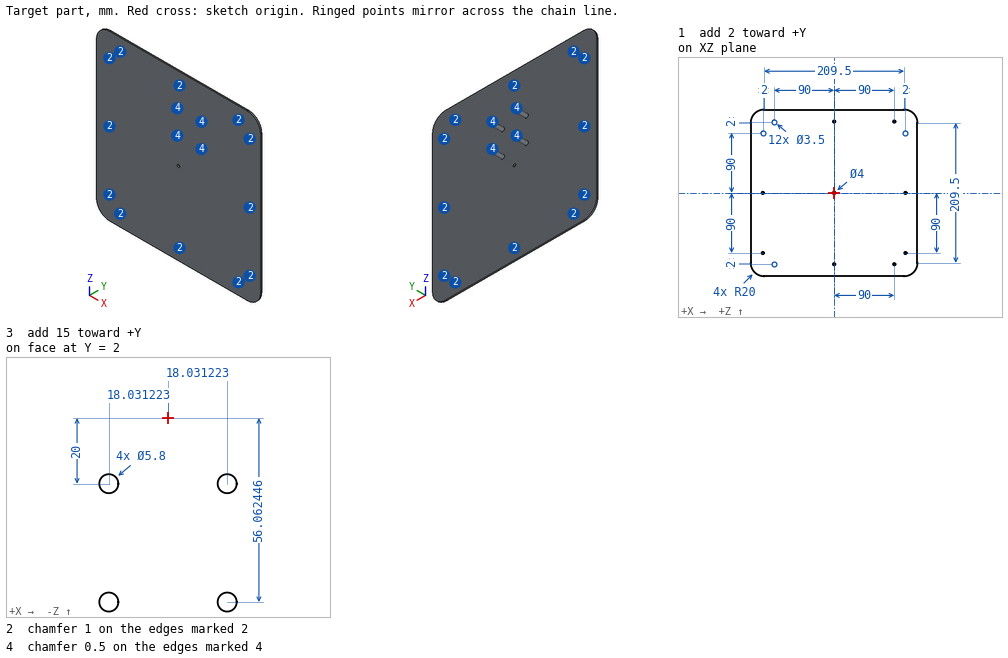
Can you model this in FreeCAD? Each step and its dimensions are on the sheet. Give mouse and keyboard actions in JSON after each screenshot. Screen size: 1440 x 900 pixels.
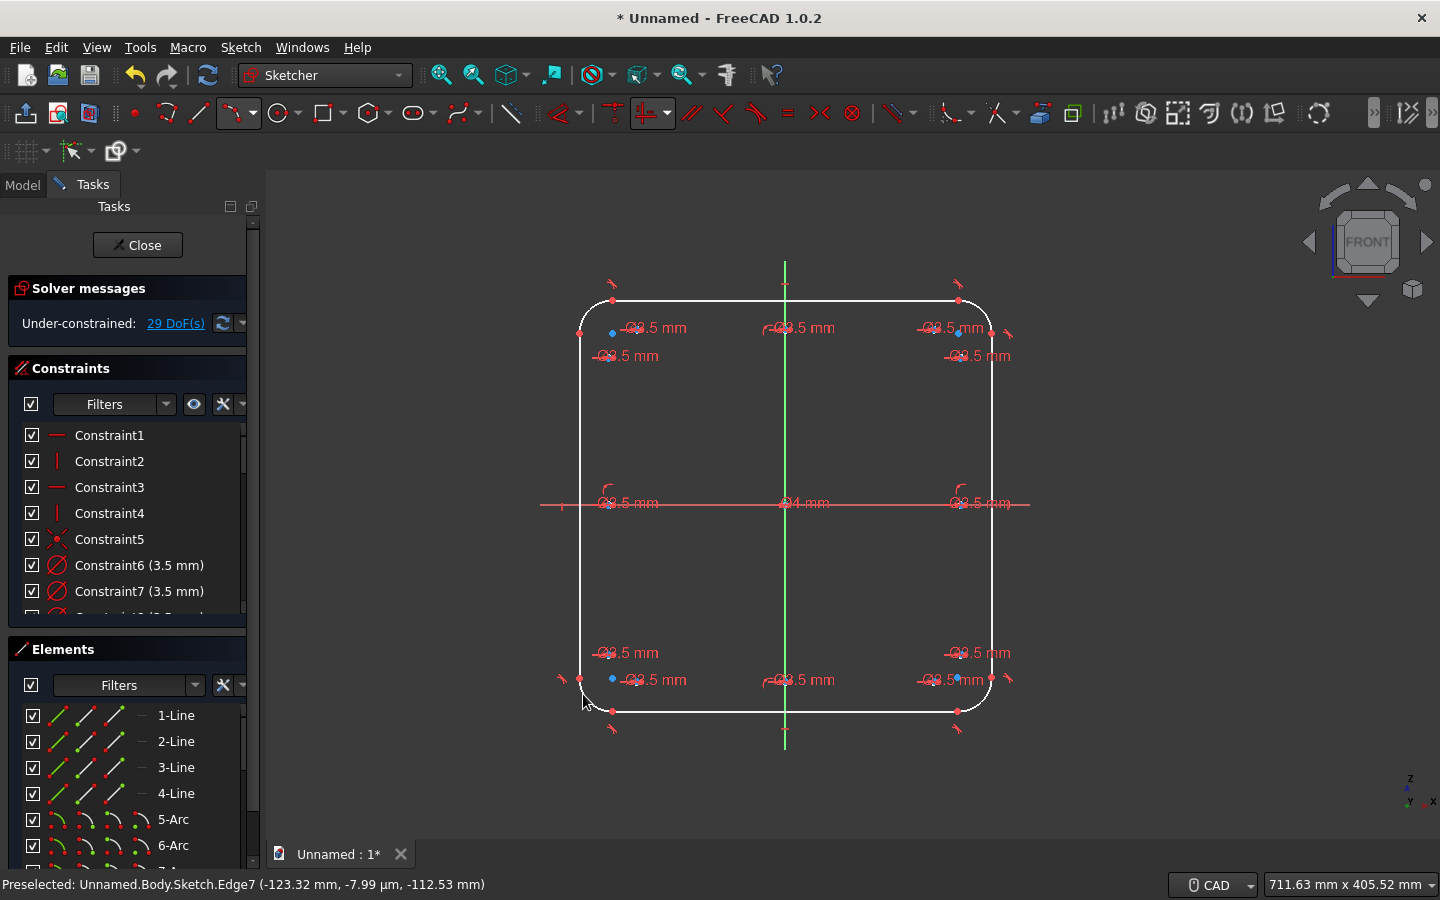
{"action": "left_click", "coordinate": [580, 575]}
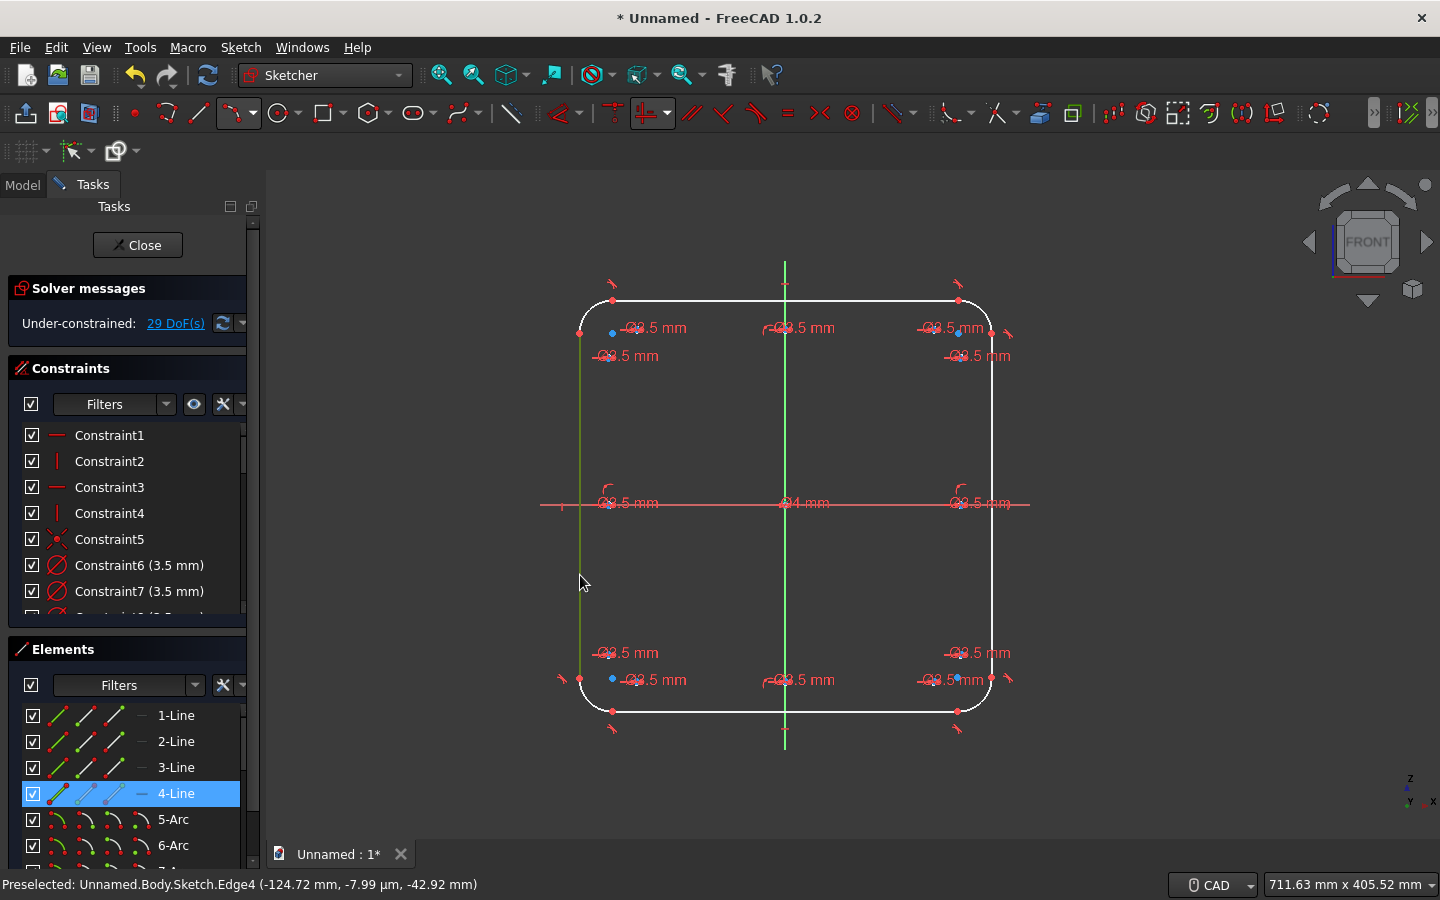
{"action": "left_click", "coordinate": [598, 304]}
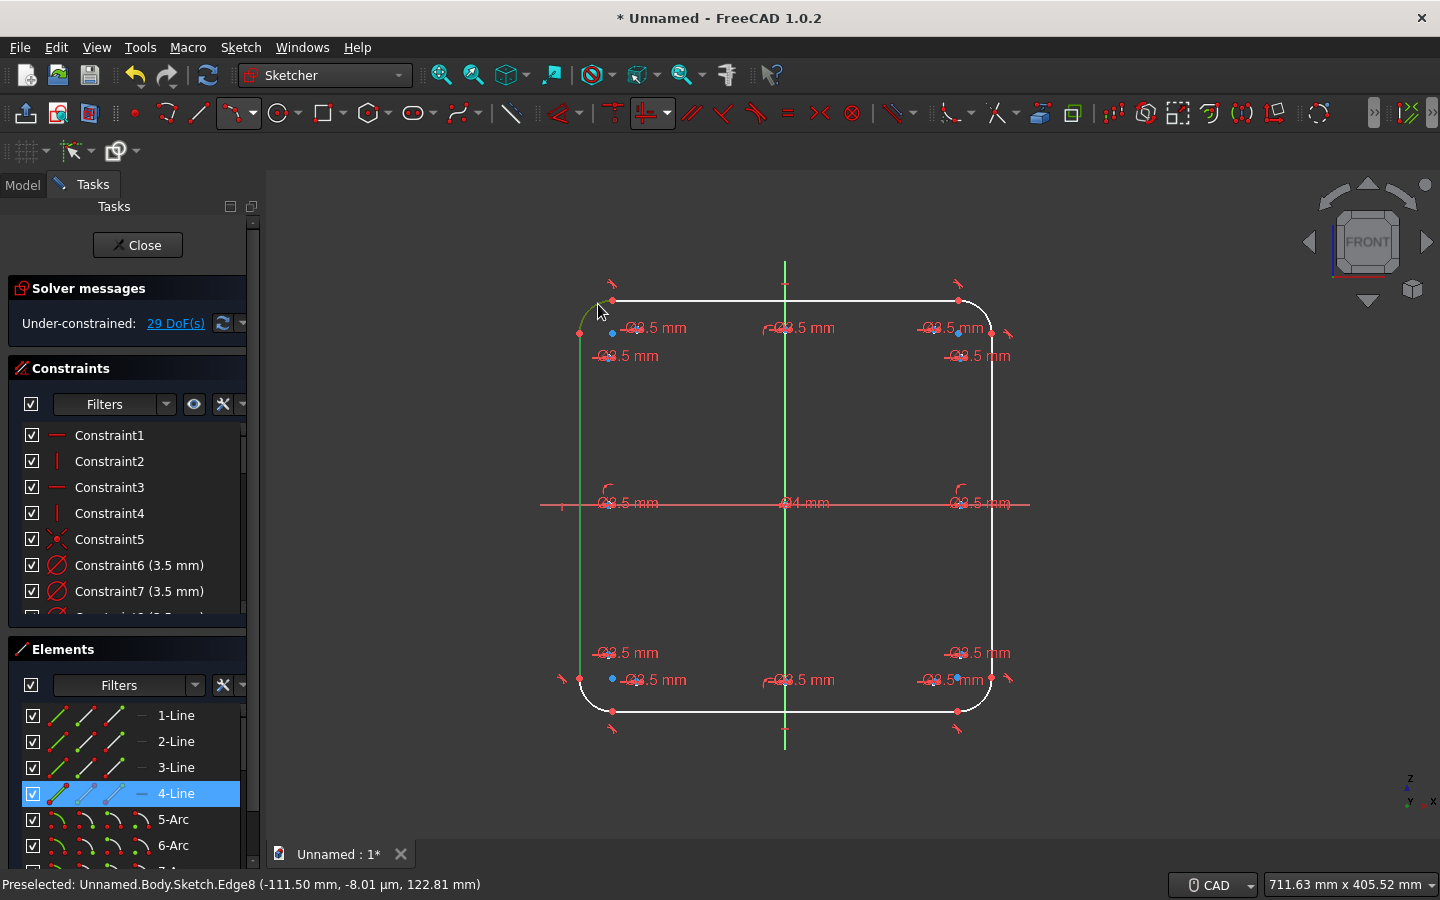
{"action": "left_click", "coordinate": [756, 114]}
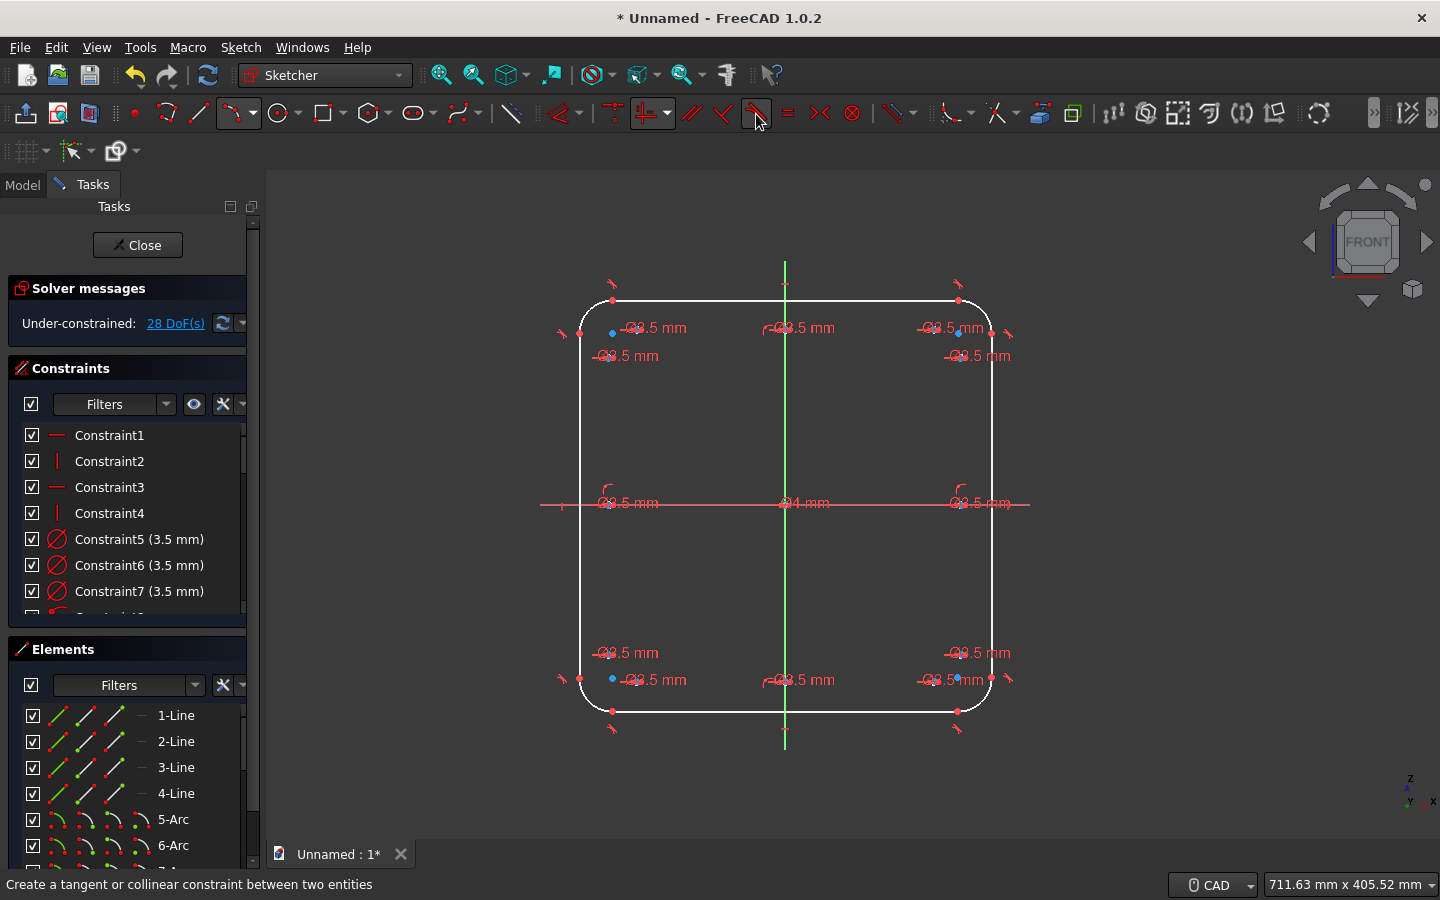
{"action": "left_click", "coordinate": [988, 319]}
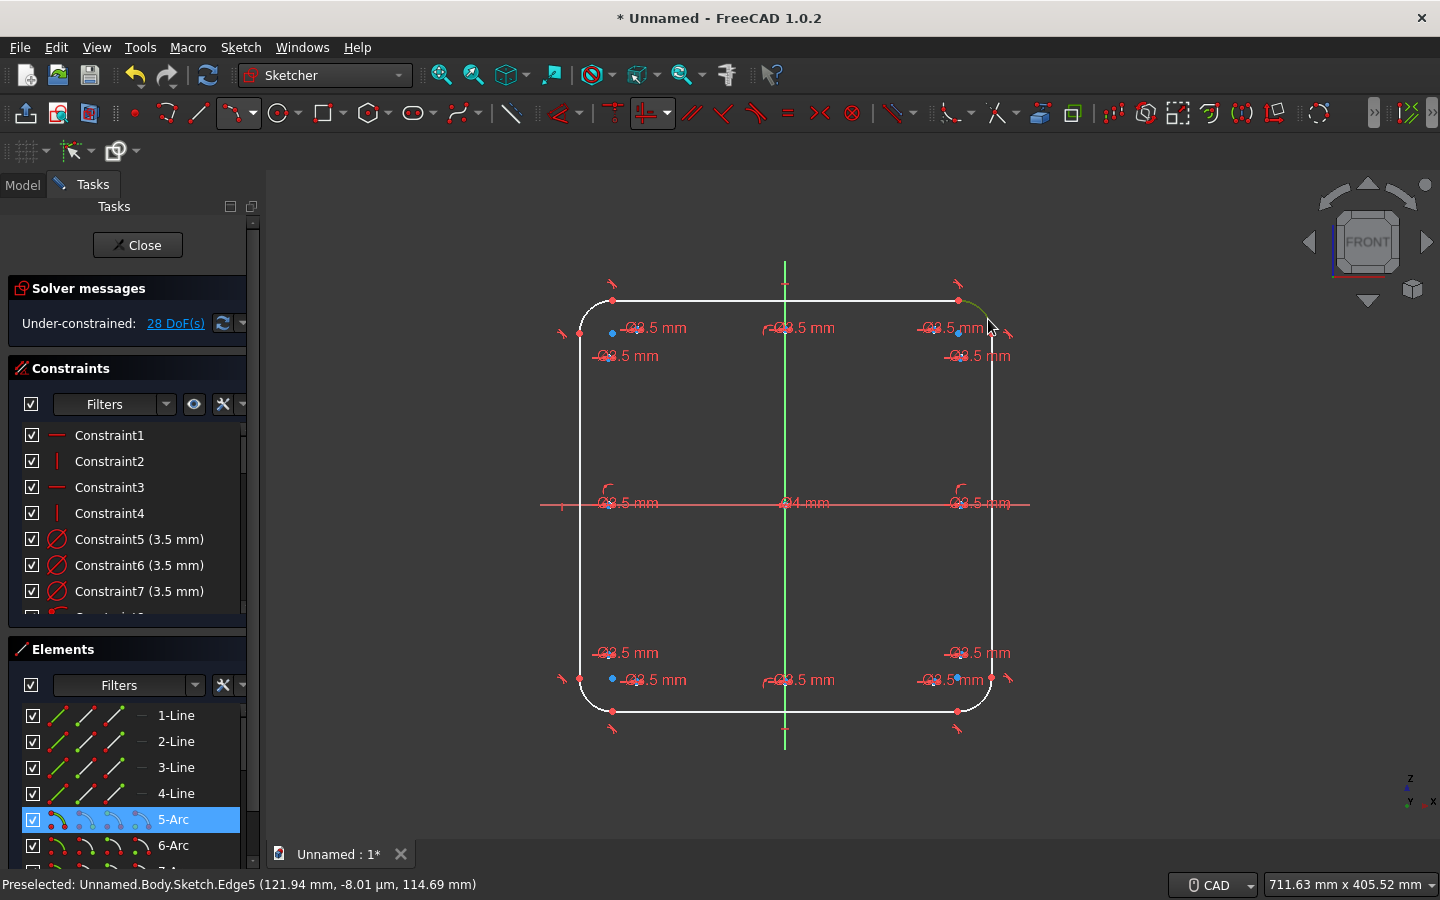
{"action": "left_click", "coordinate": [973, 708]}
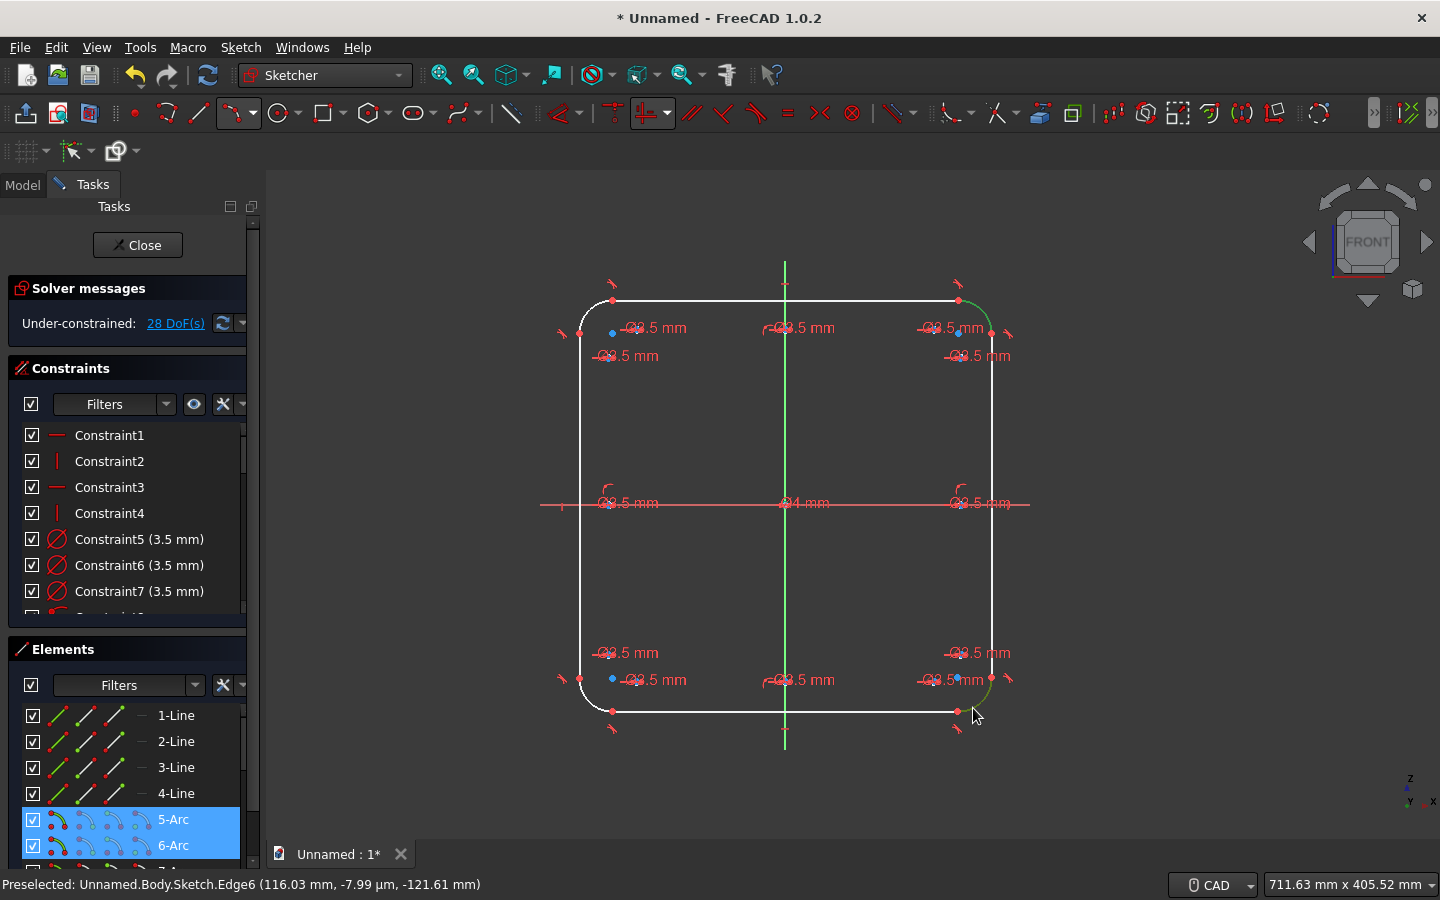
{"action": "left_click", "coordinate": [583, 694]}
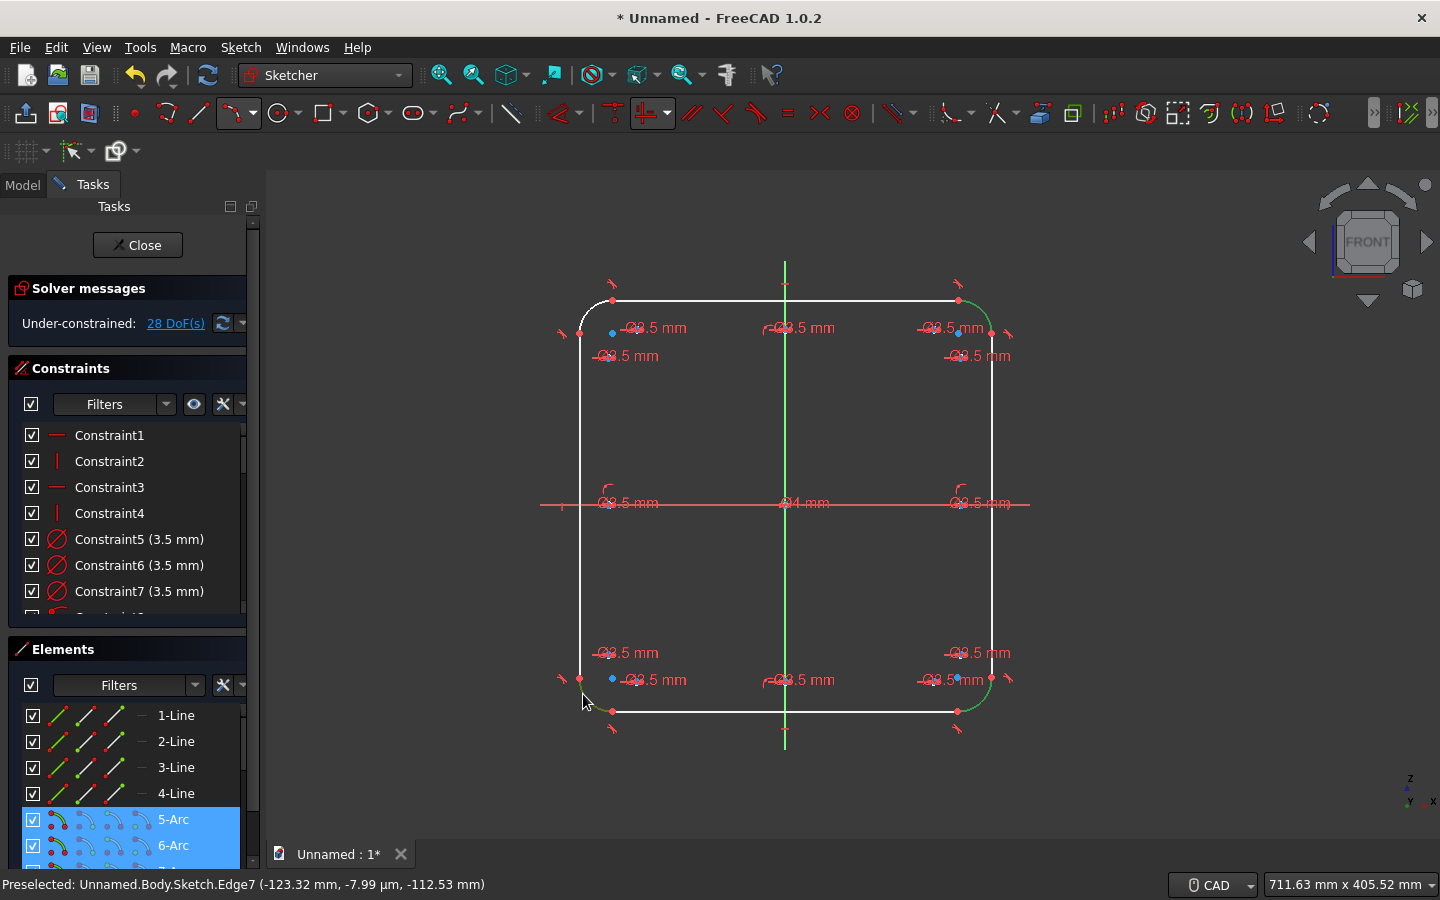
{"action": "left_click", "coordinate": [598, 304]}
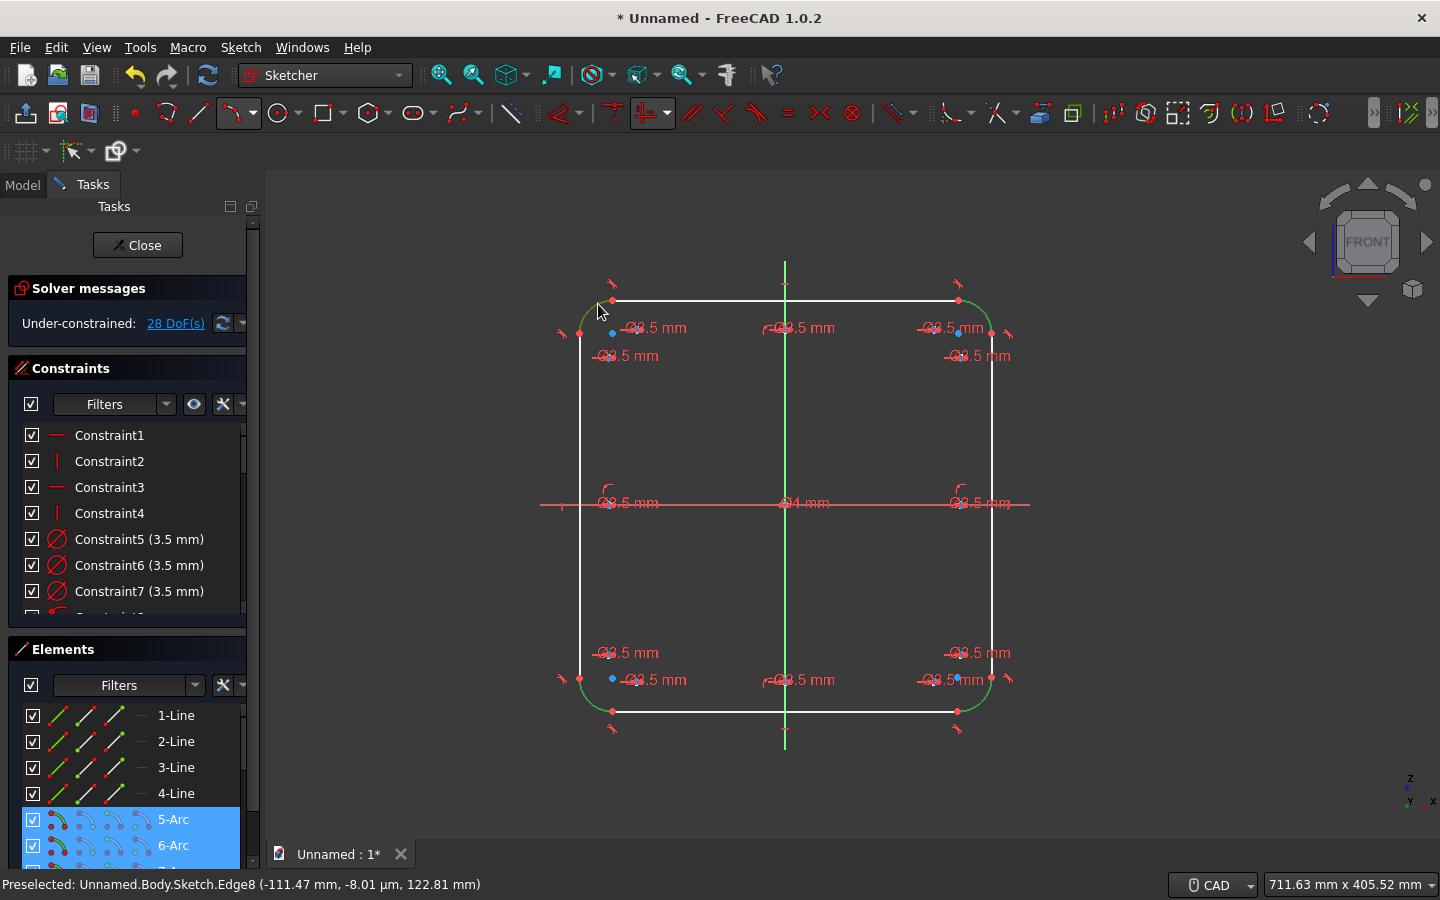
{"action": "key", "text": "e"}